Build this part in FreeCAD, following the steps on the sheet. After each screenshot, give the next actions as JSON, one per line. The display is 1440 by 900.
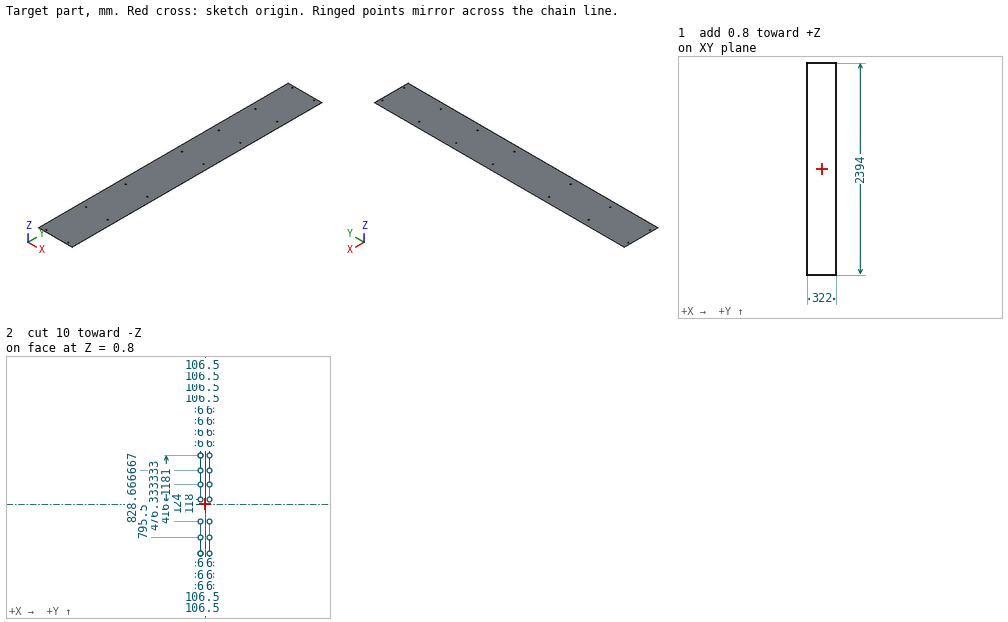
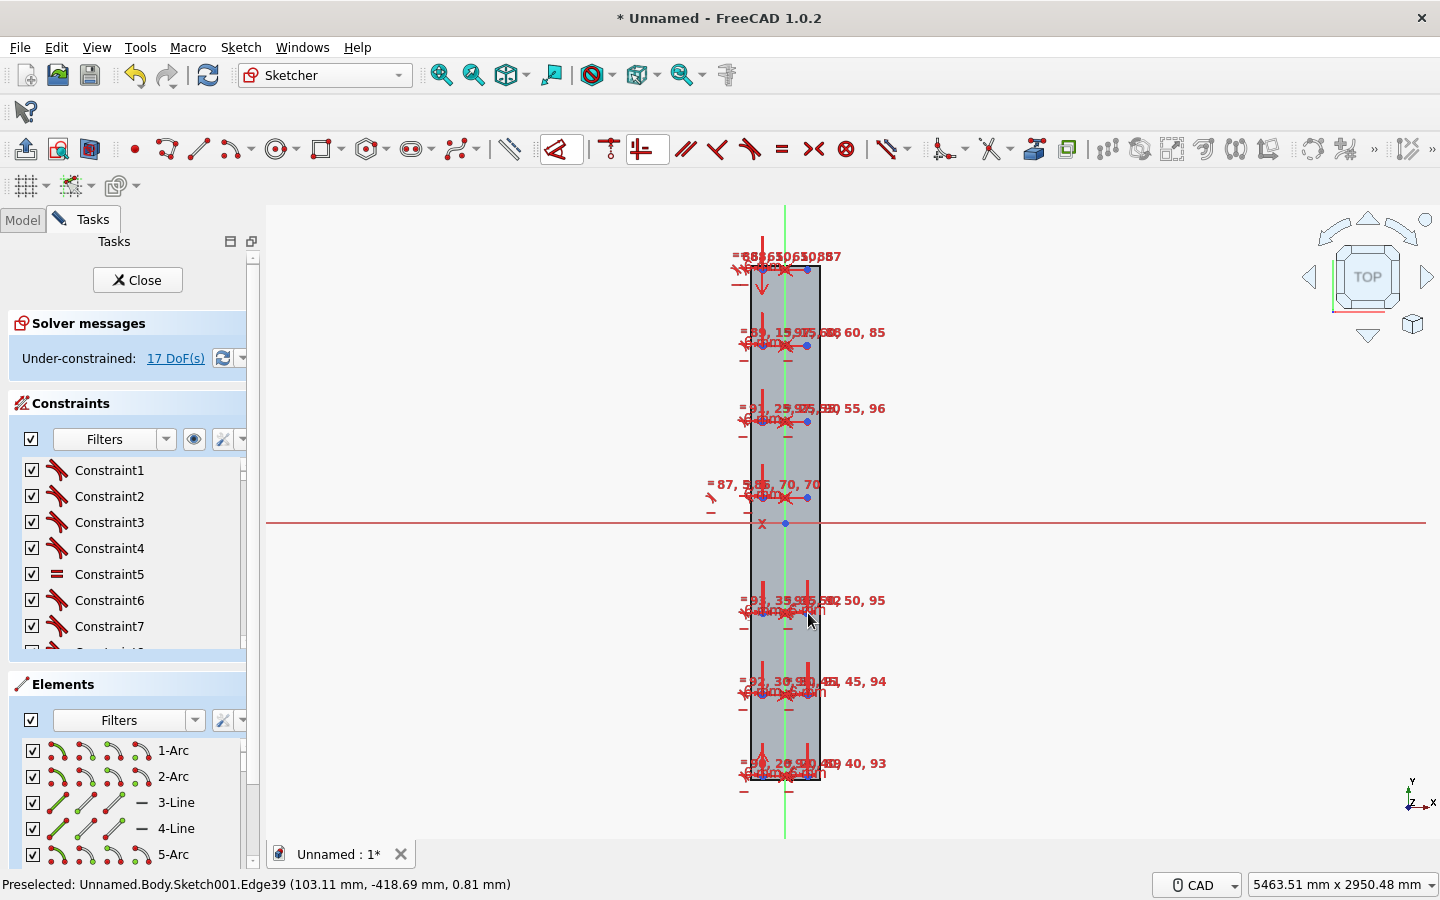
{"action": "scroll", "coordinate": [807, 422], "scroll_direction": "up", "scroll_amount": 18}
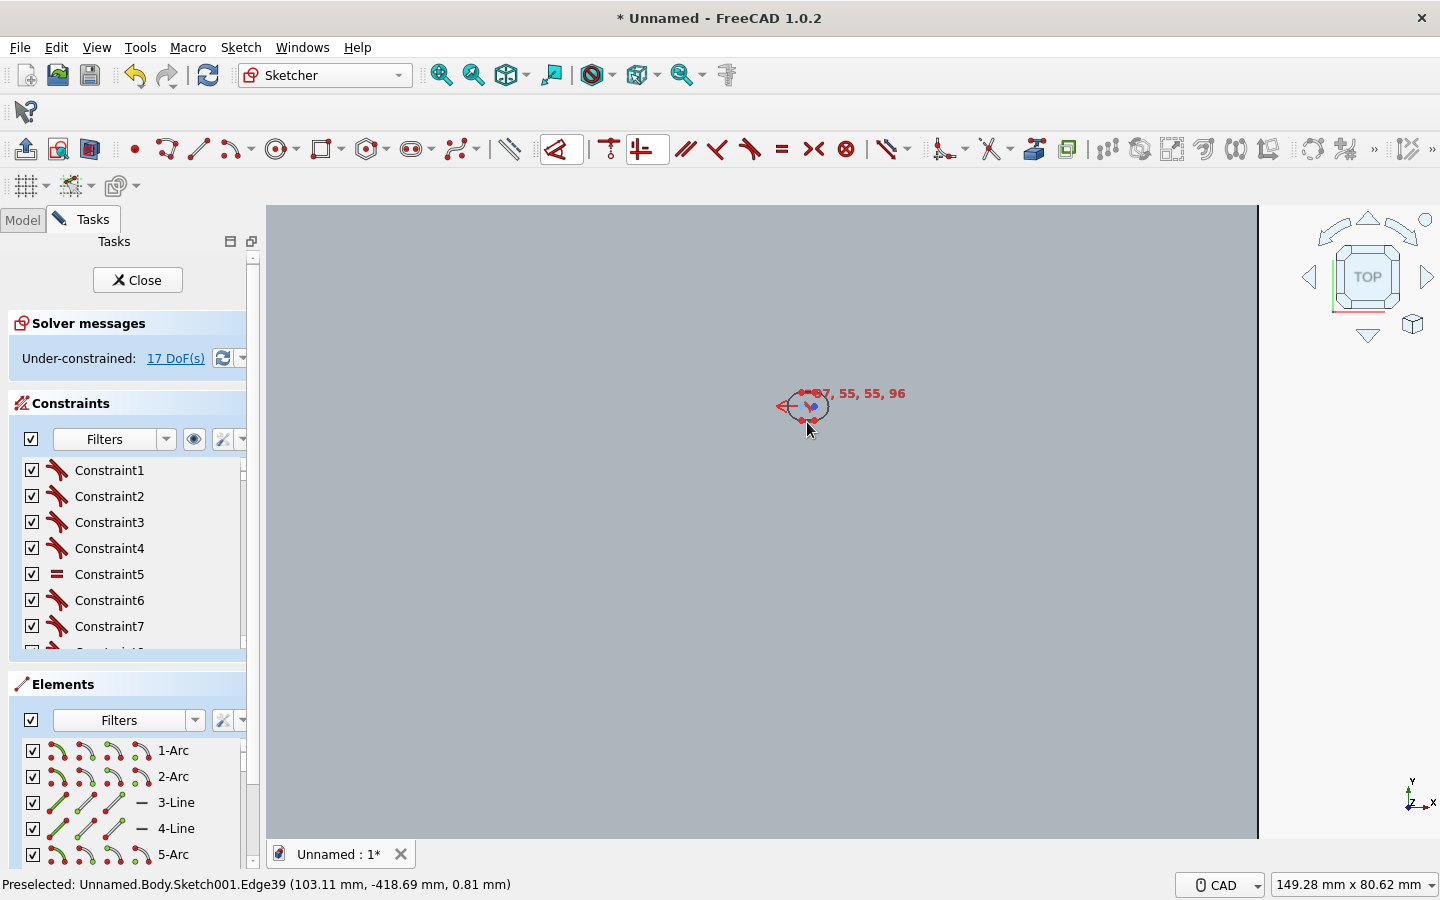
{"action": "scroll", "coordinate": [808, 392], "scroll_direction": "up", "scroll_amount": 4}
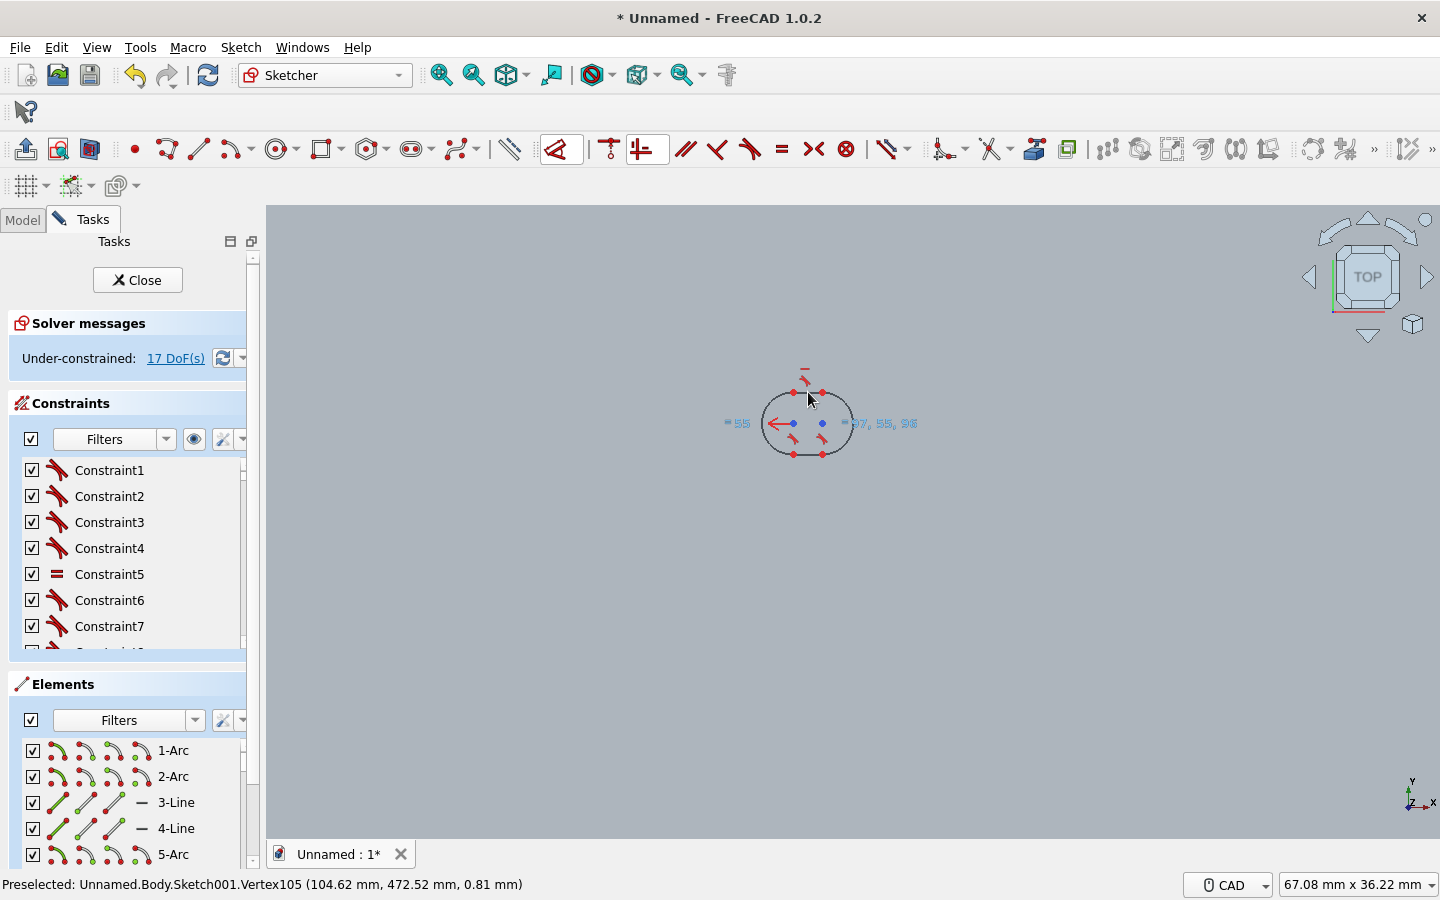
{"action": "left_click", "coordinate": [808, 393]}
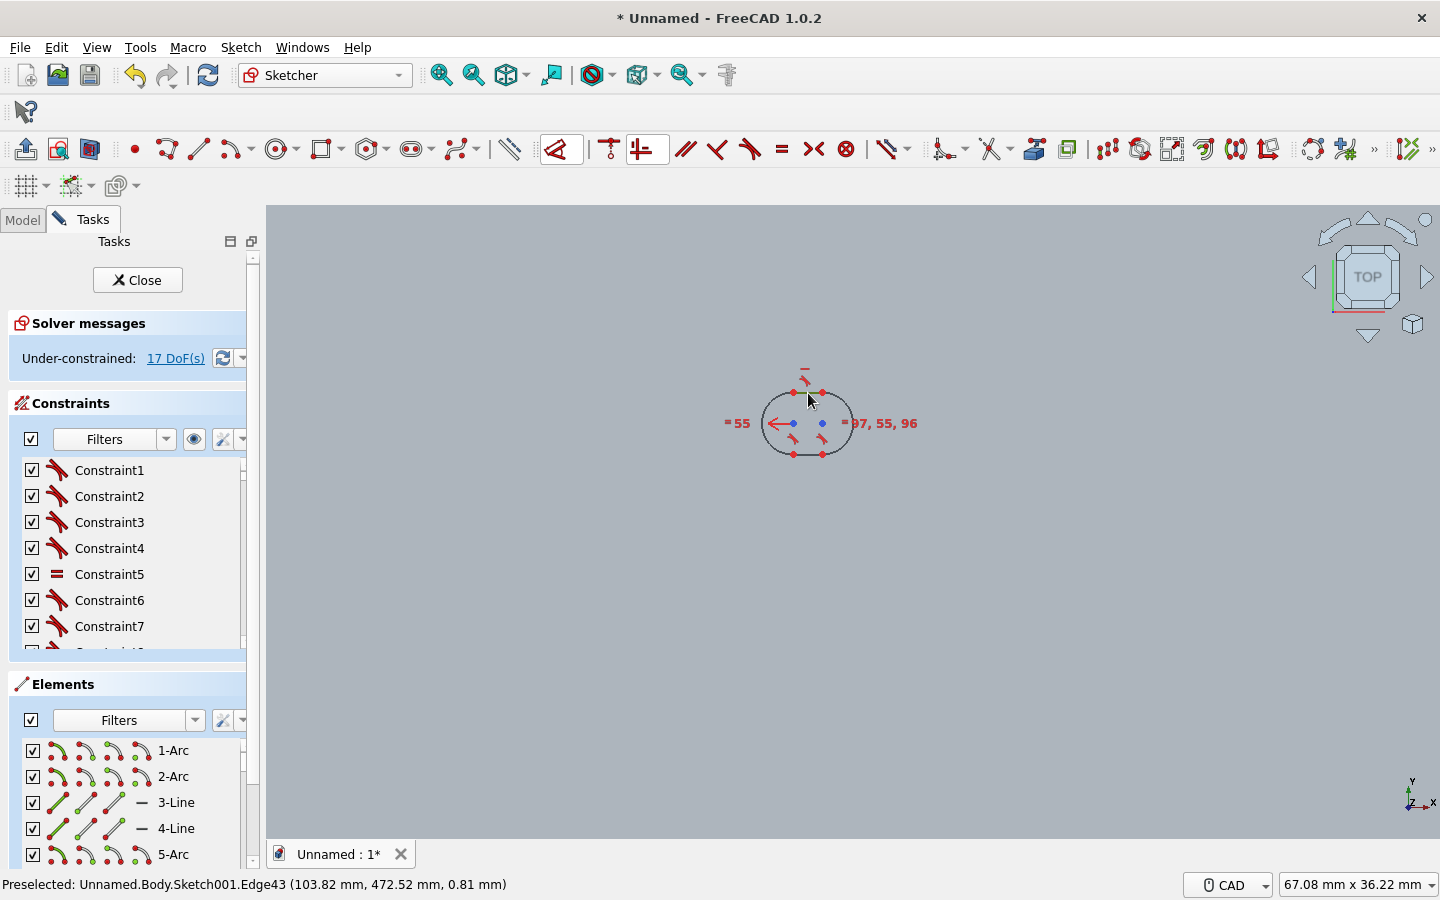
{"action": "key", "text": "l"}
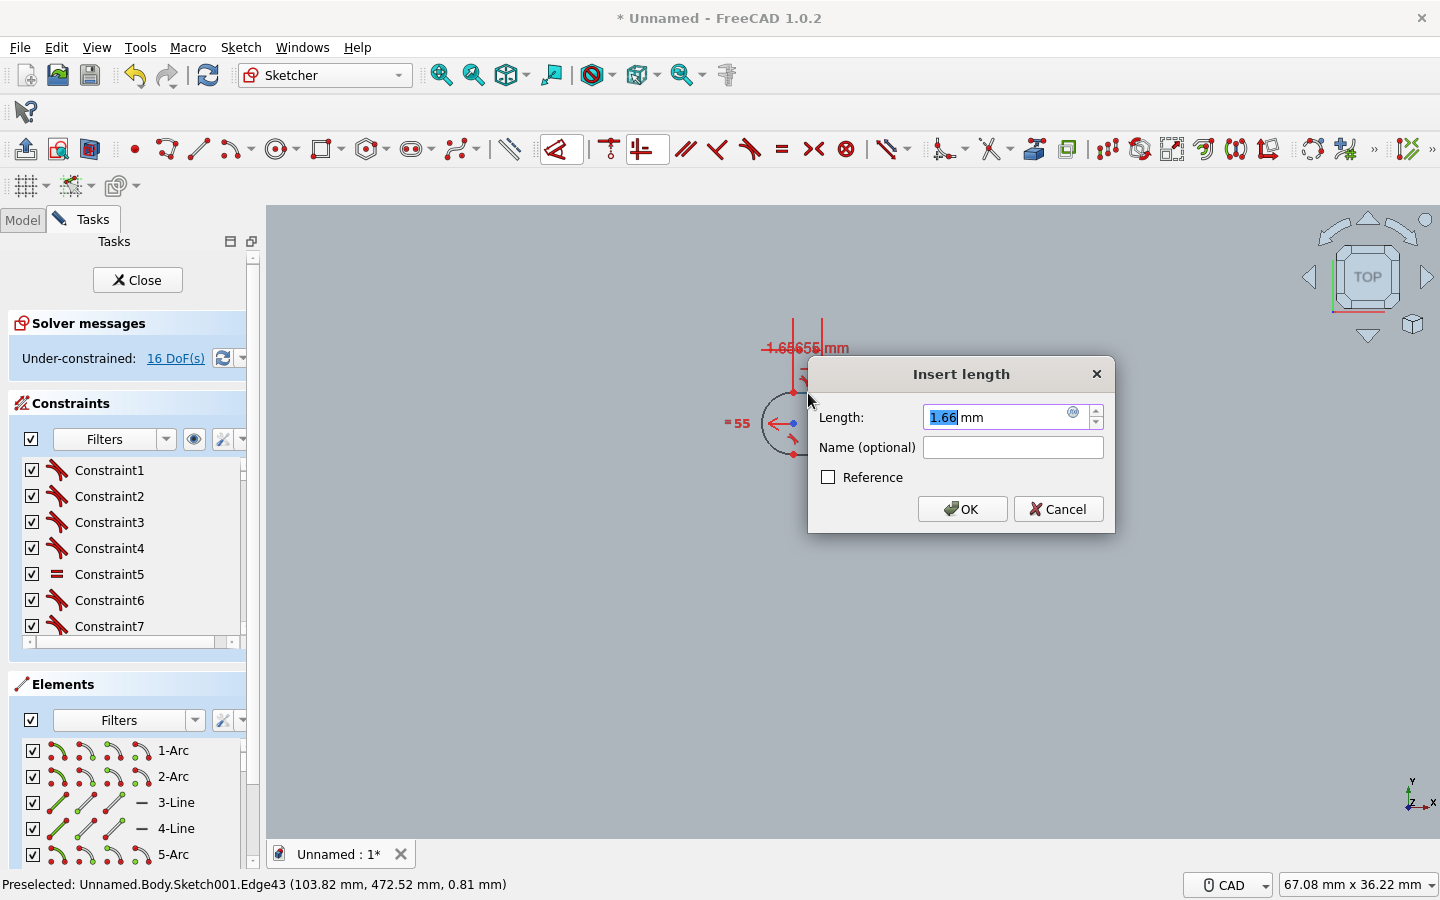
{"action": "type", "text": "6"}
{"action": "key", "text": "Return"}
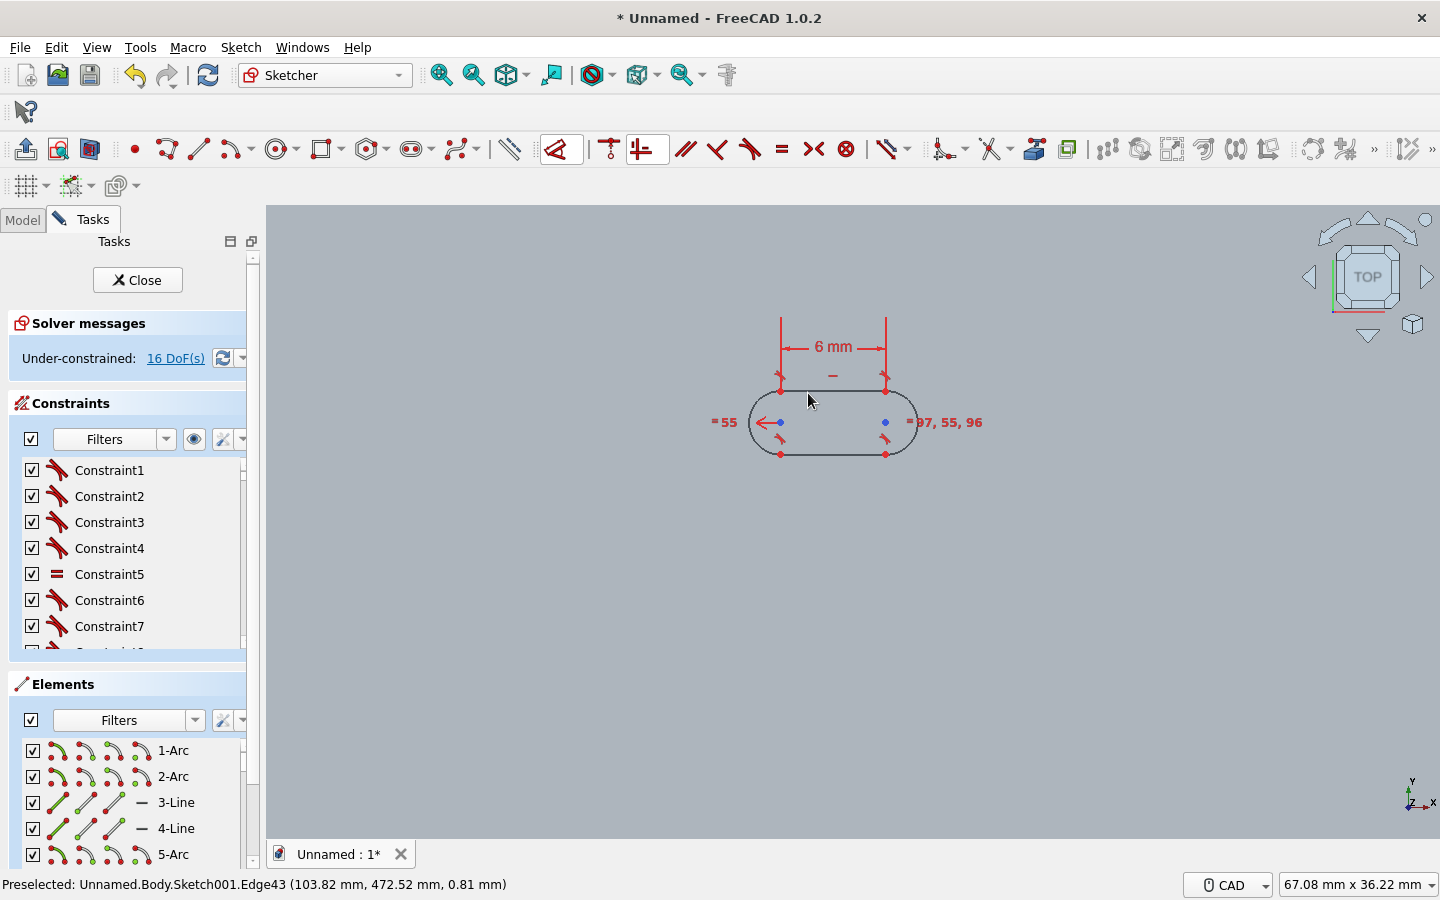
{"action": "scroll", "coordinate": [784, 522], "scroll_direction": "down", "scroll_amount": 15}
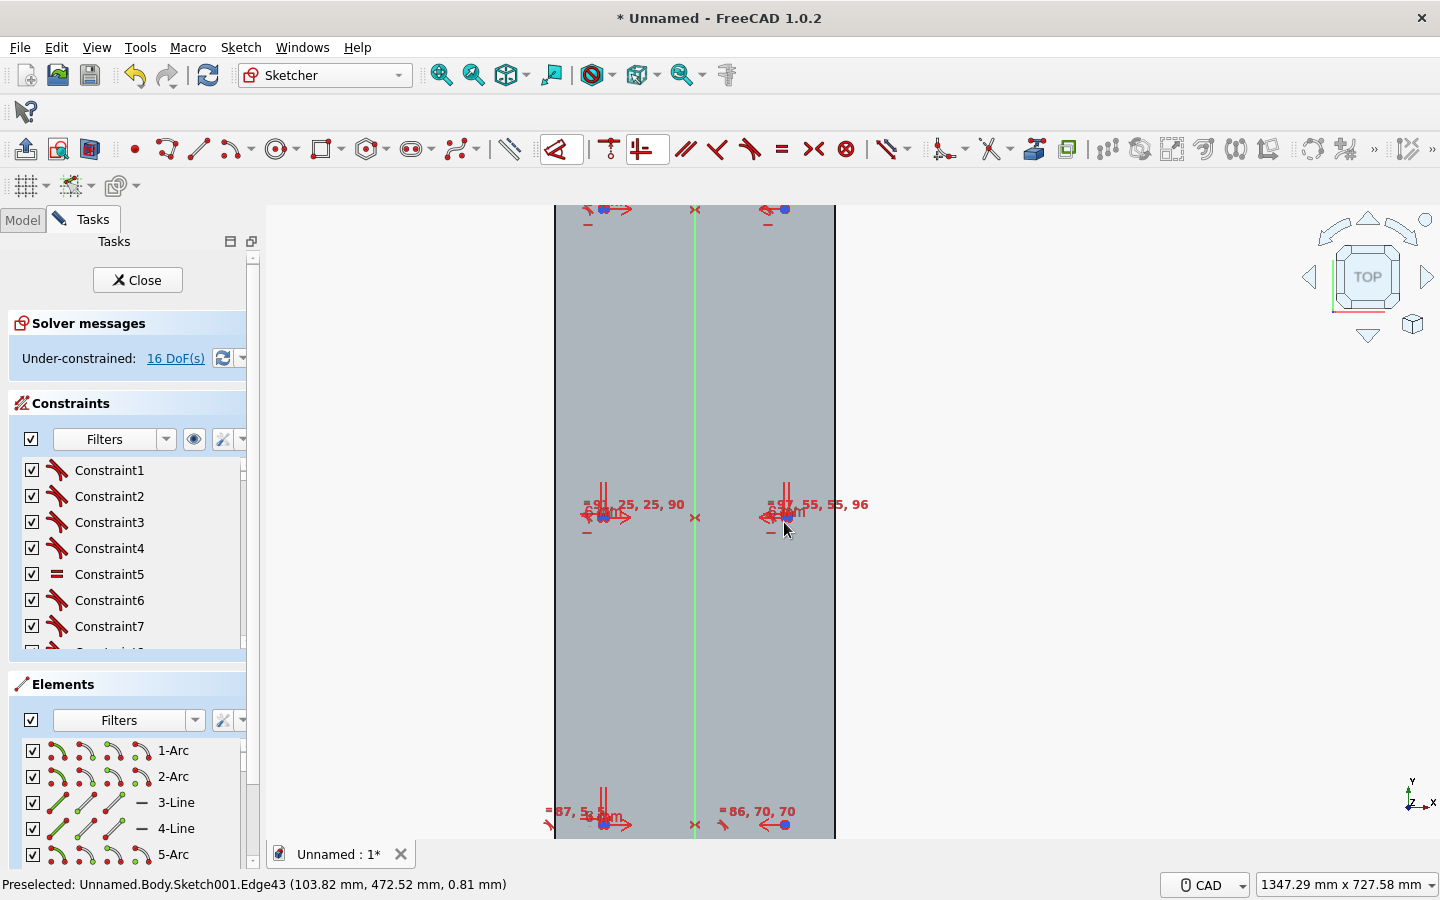
{"action": "scroll", "coordinate": [807, 419], "scroll_direction": "down", "scroll_amount": 8}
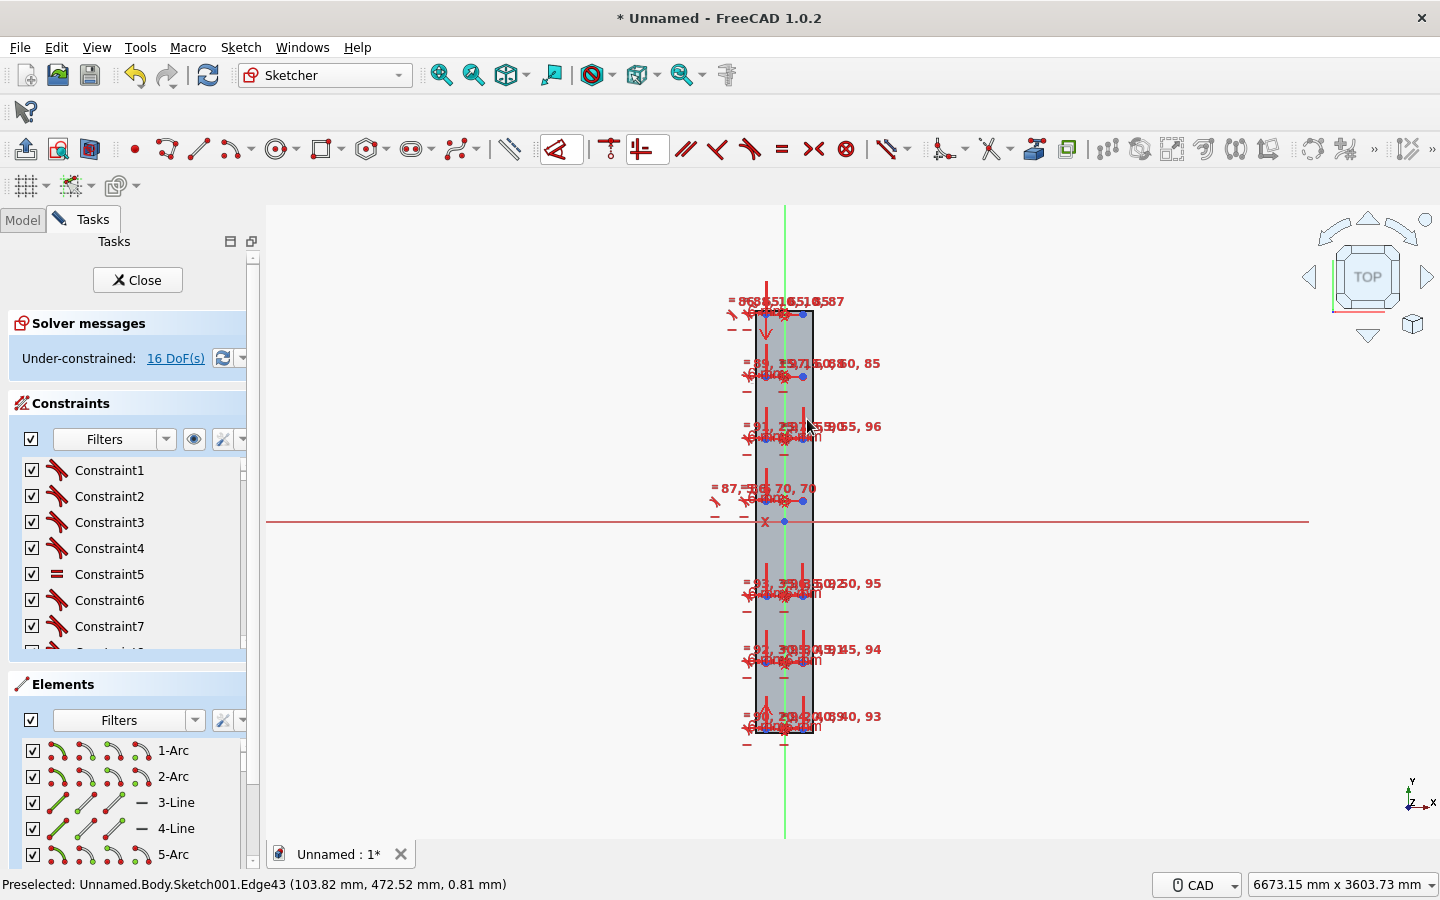
{"action": "scroll", "coordinate": [803, 377], "scroll_direction": "up", "scroll_amount": 19}